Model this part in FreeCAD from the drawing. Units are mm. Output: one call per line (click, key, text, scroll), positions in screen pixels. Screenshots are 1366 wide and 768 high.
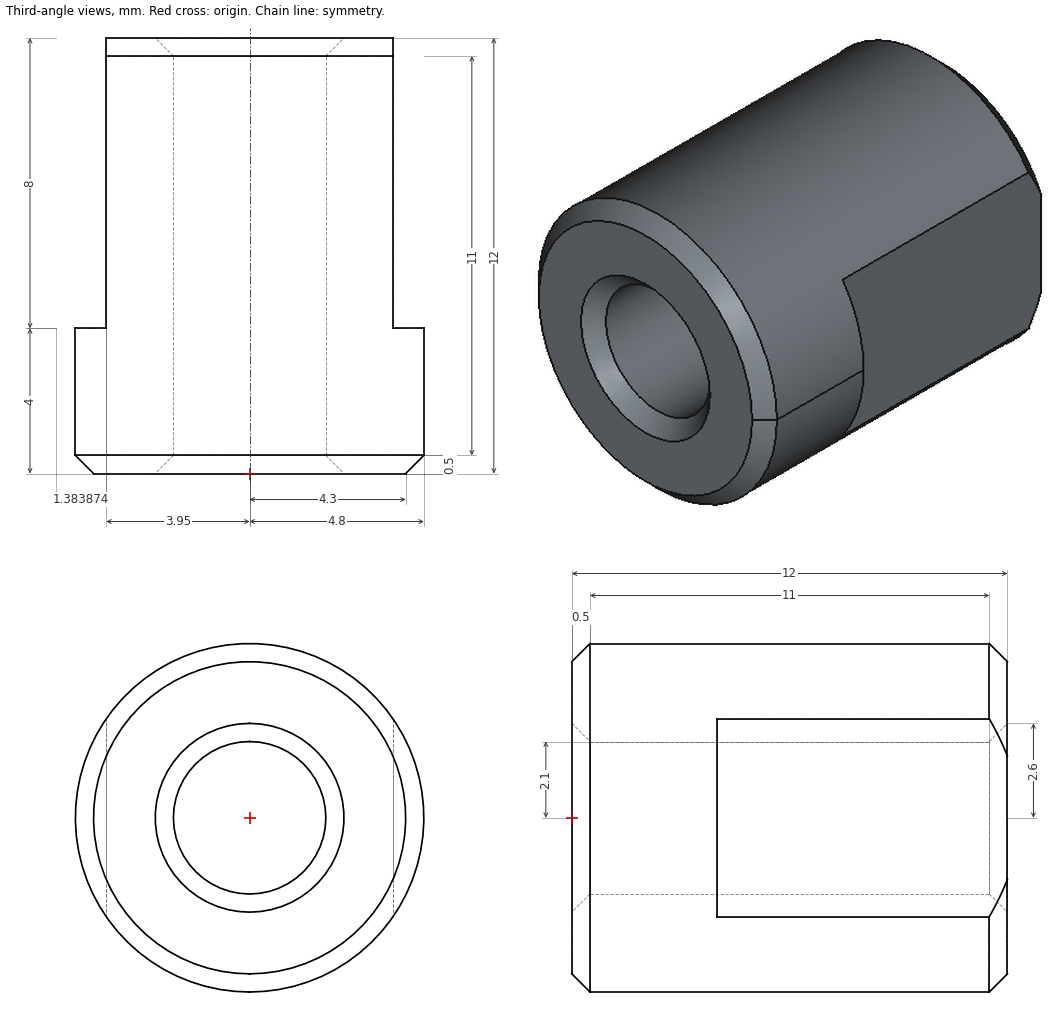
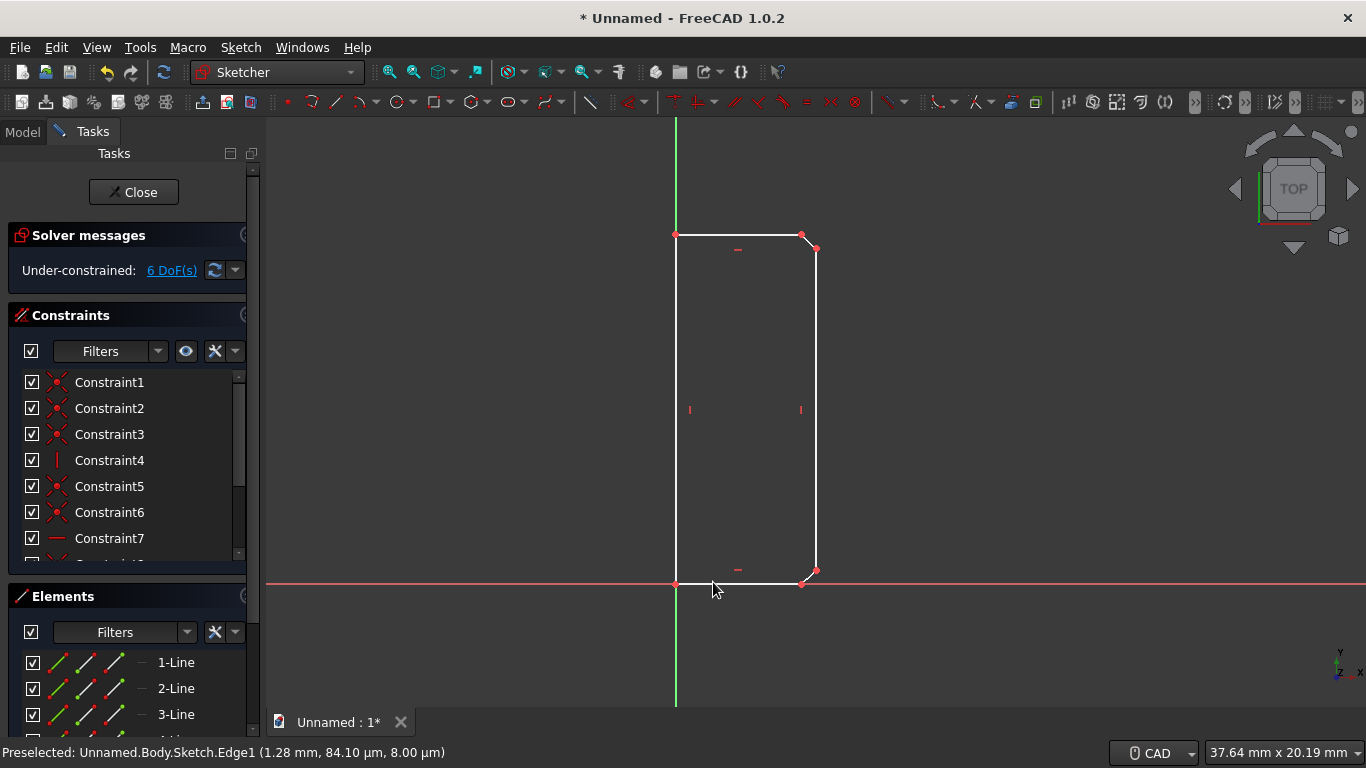
click(816, 474)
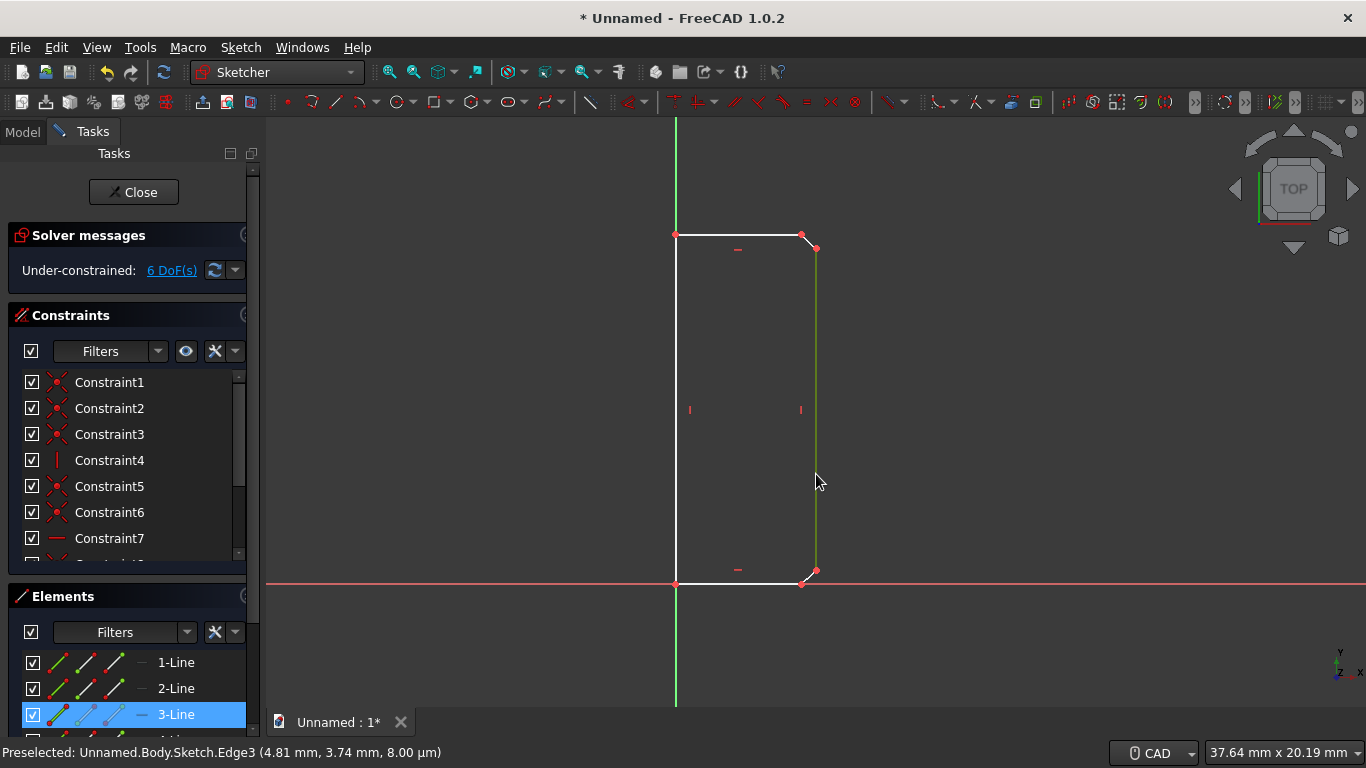
key(i)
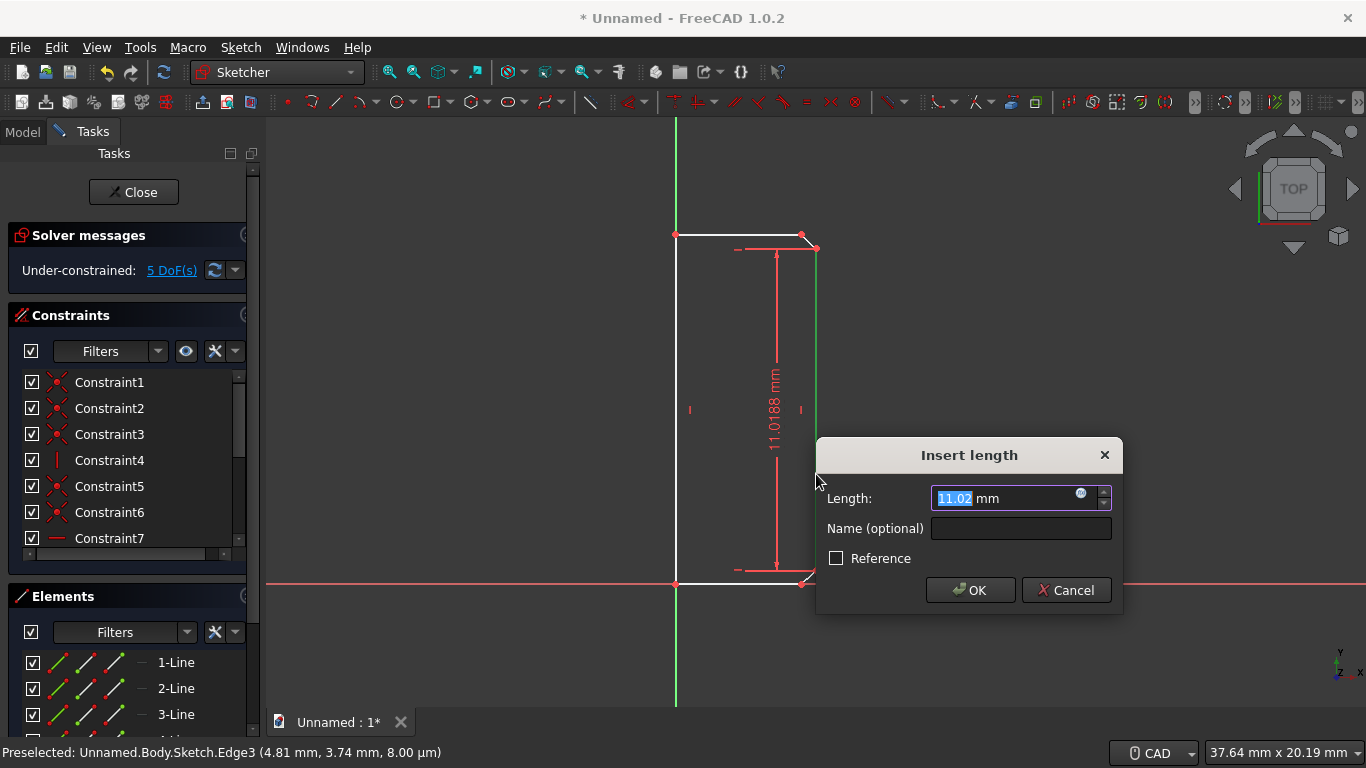
text(11)
key(Return)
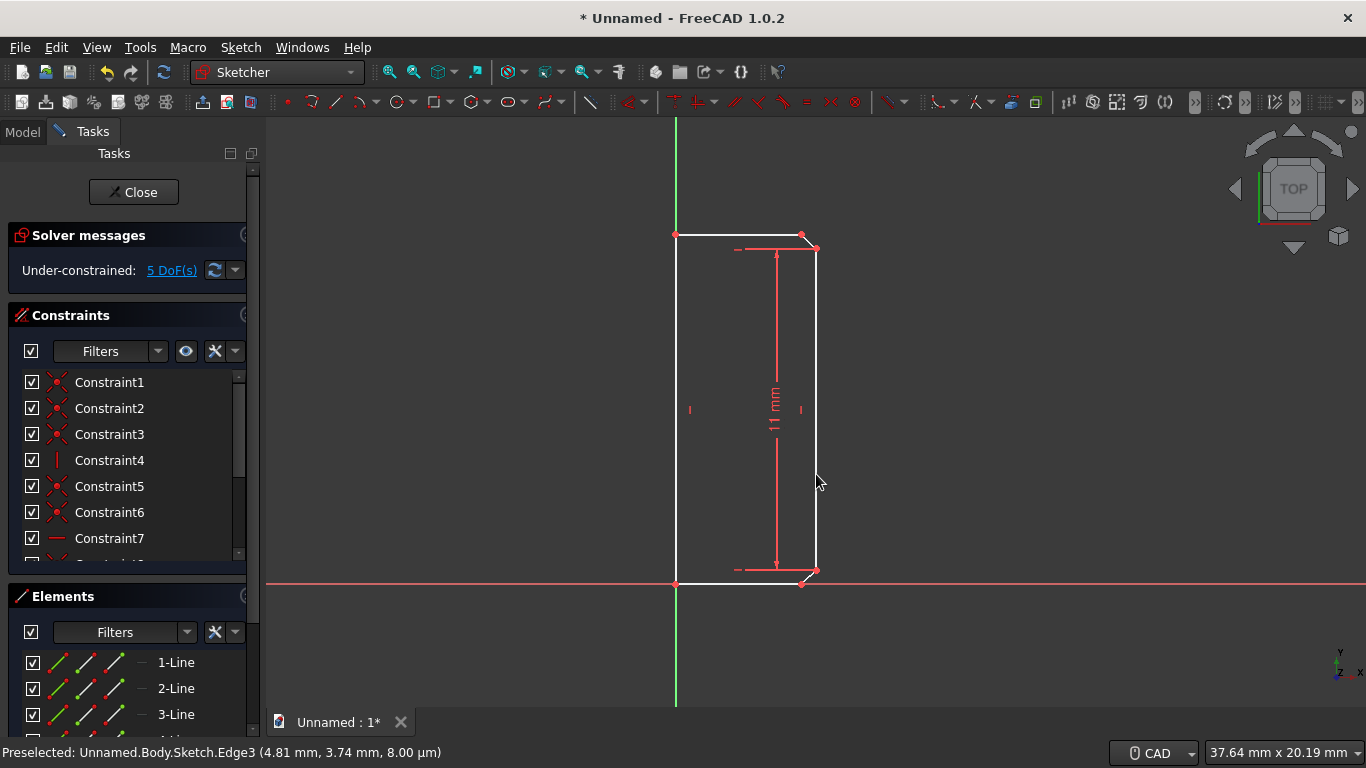
click(676, 340)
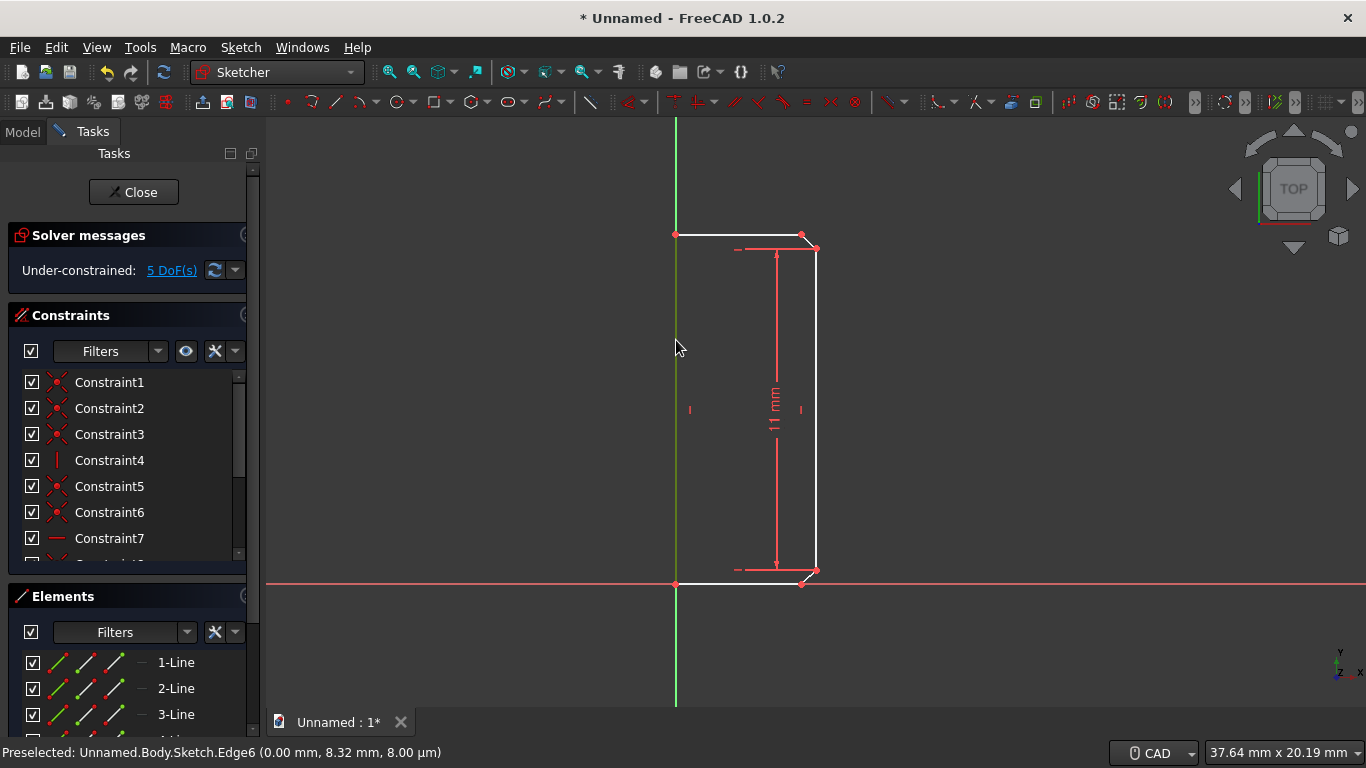
click(646, 102)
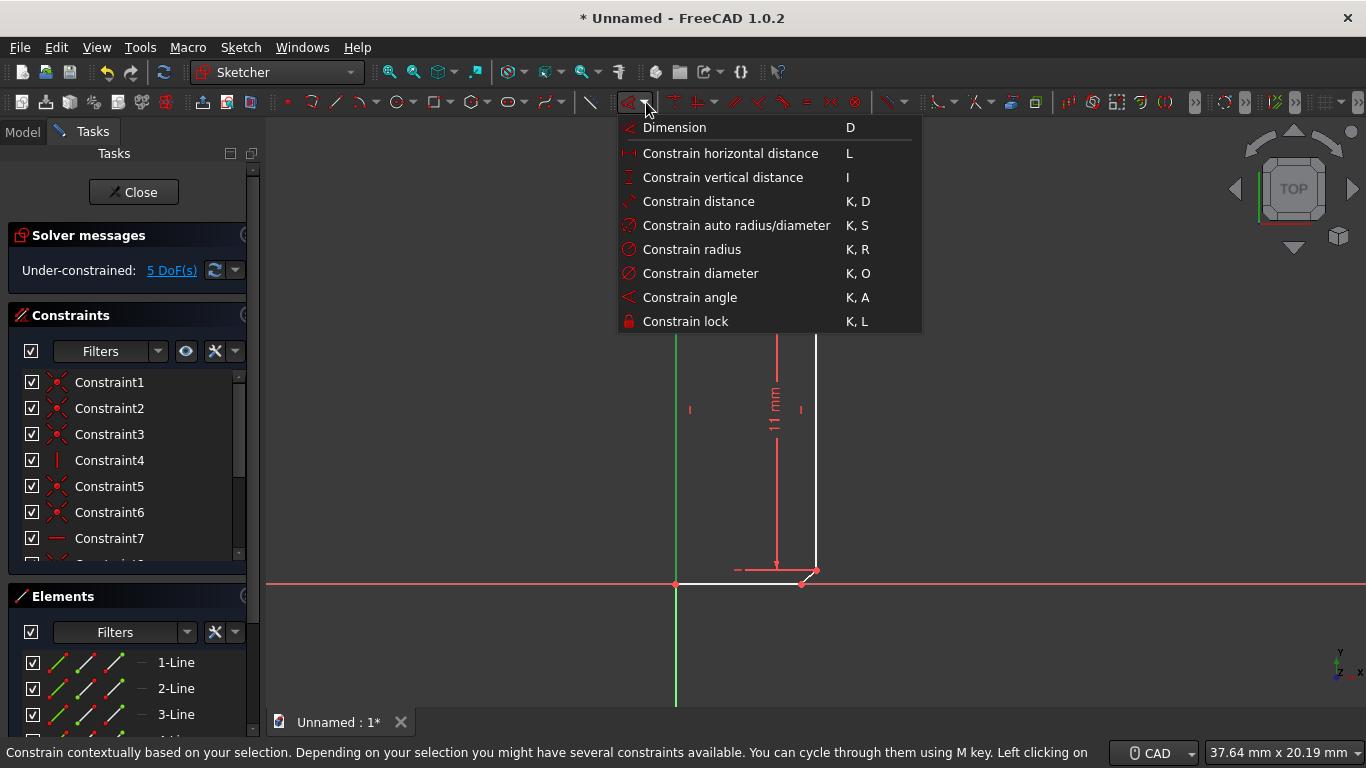
click(770, 177)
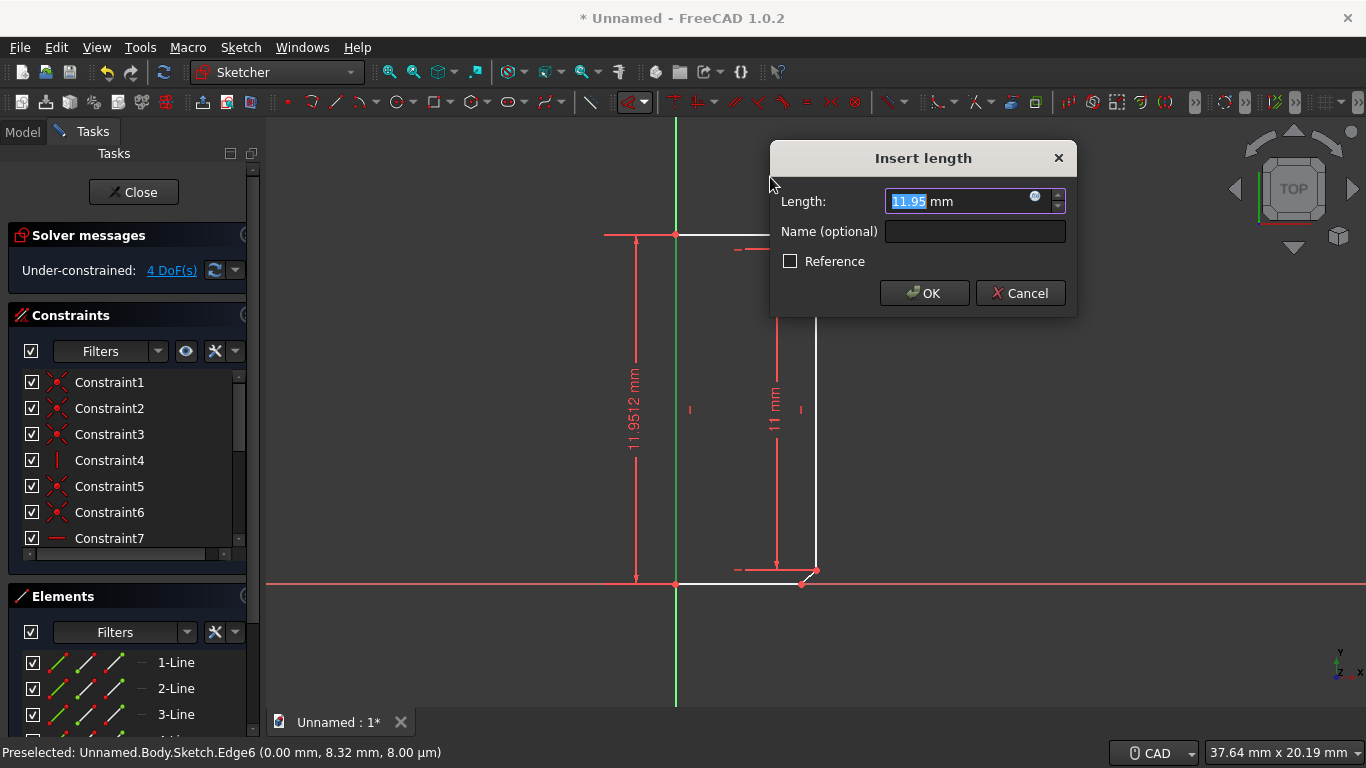
text(12)
key(Return)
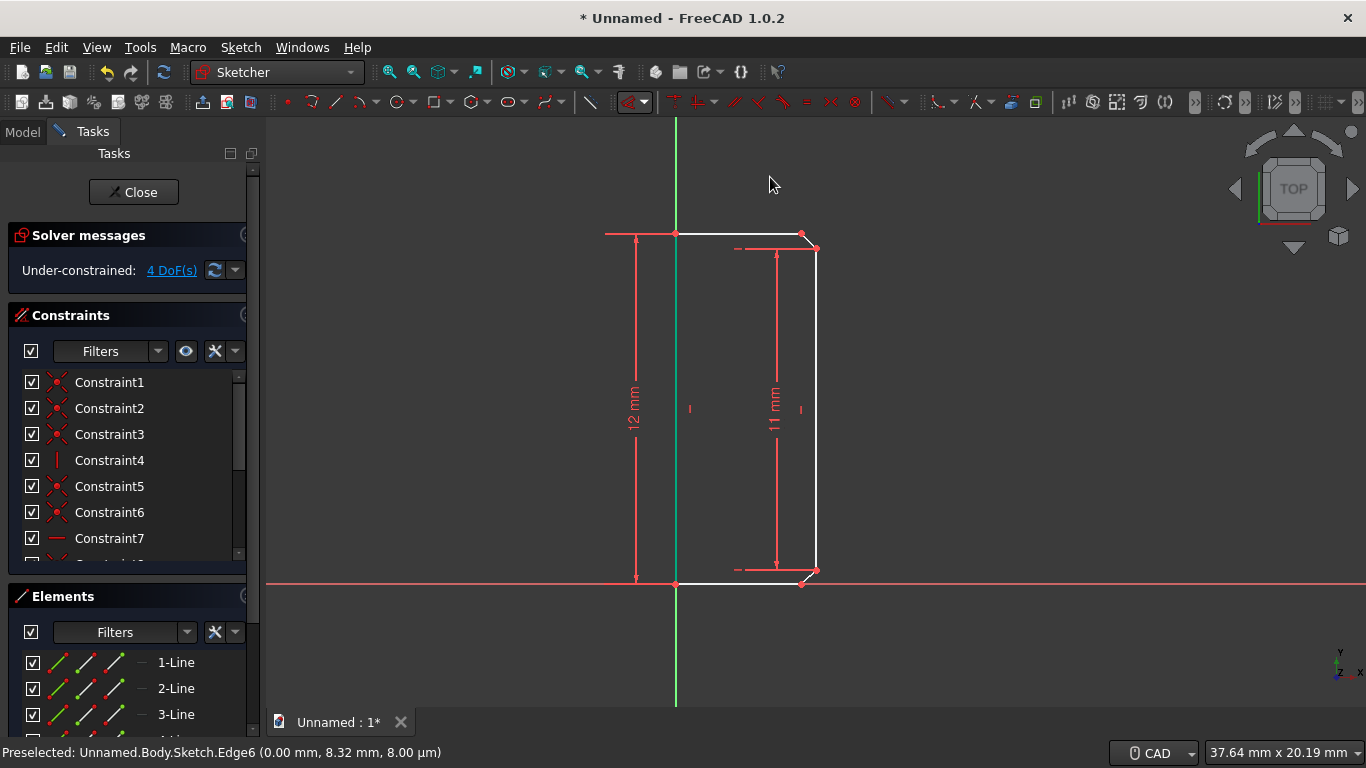
click(713, 584)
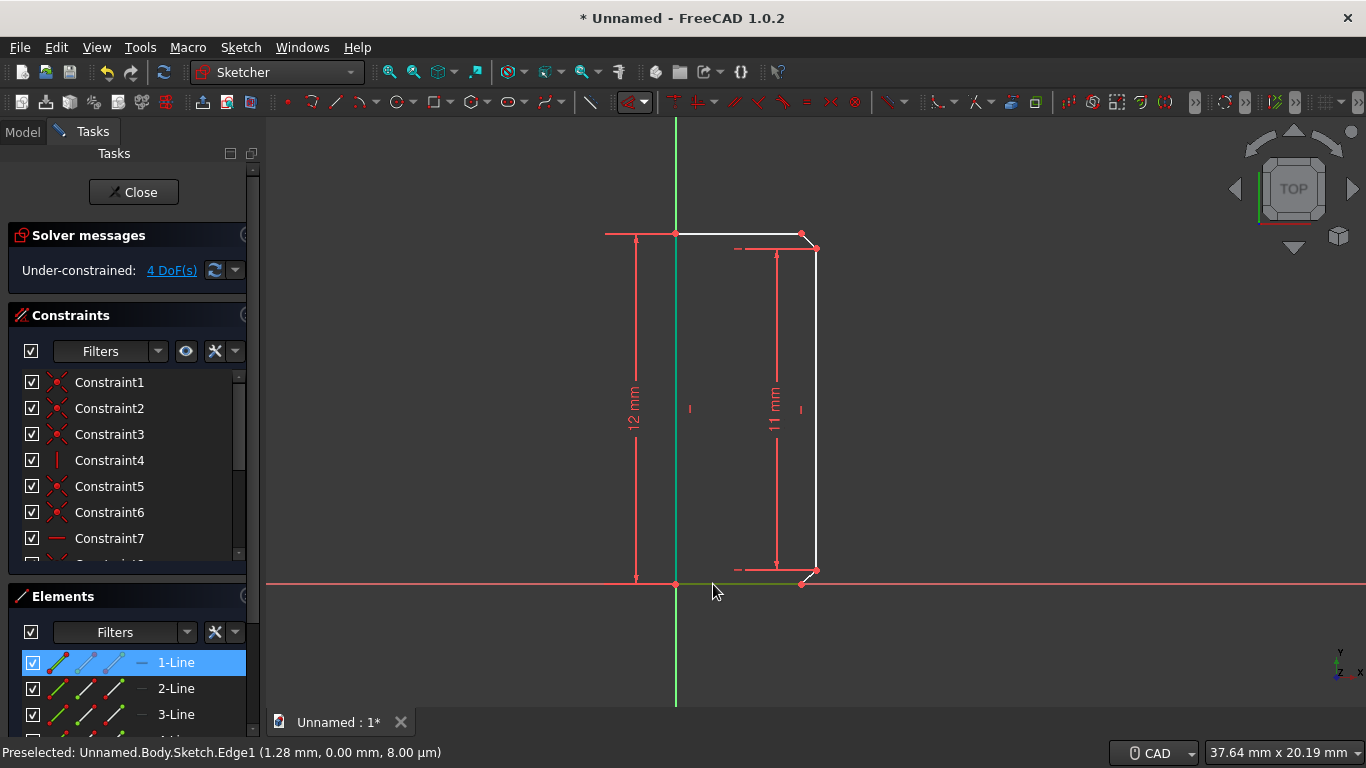
click(646, 102)